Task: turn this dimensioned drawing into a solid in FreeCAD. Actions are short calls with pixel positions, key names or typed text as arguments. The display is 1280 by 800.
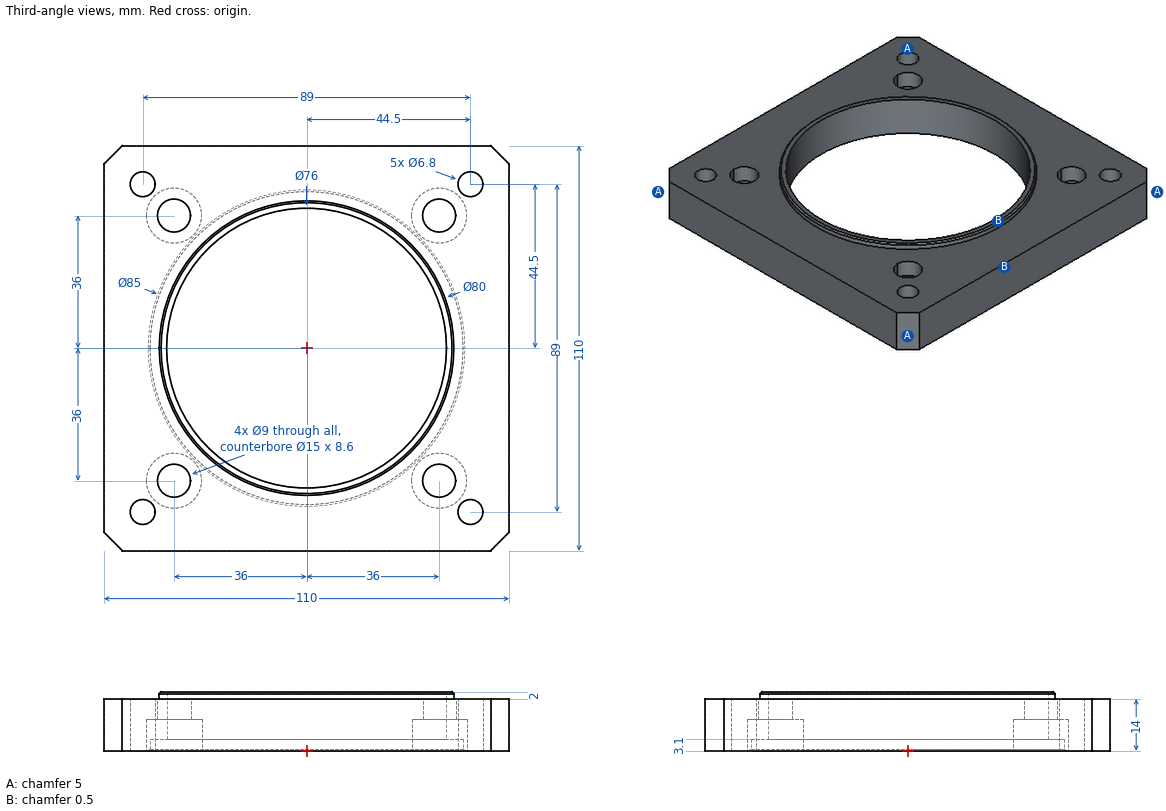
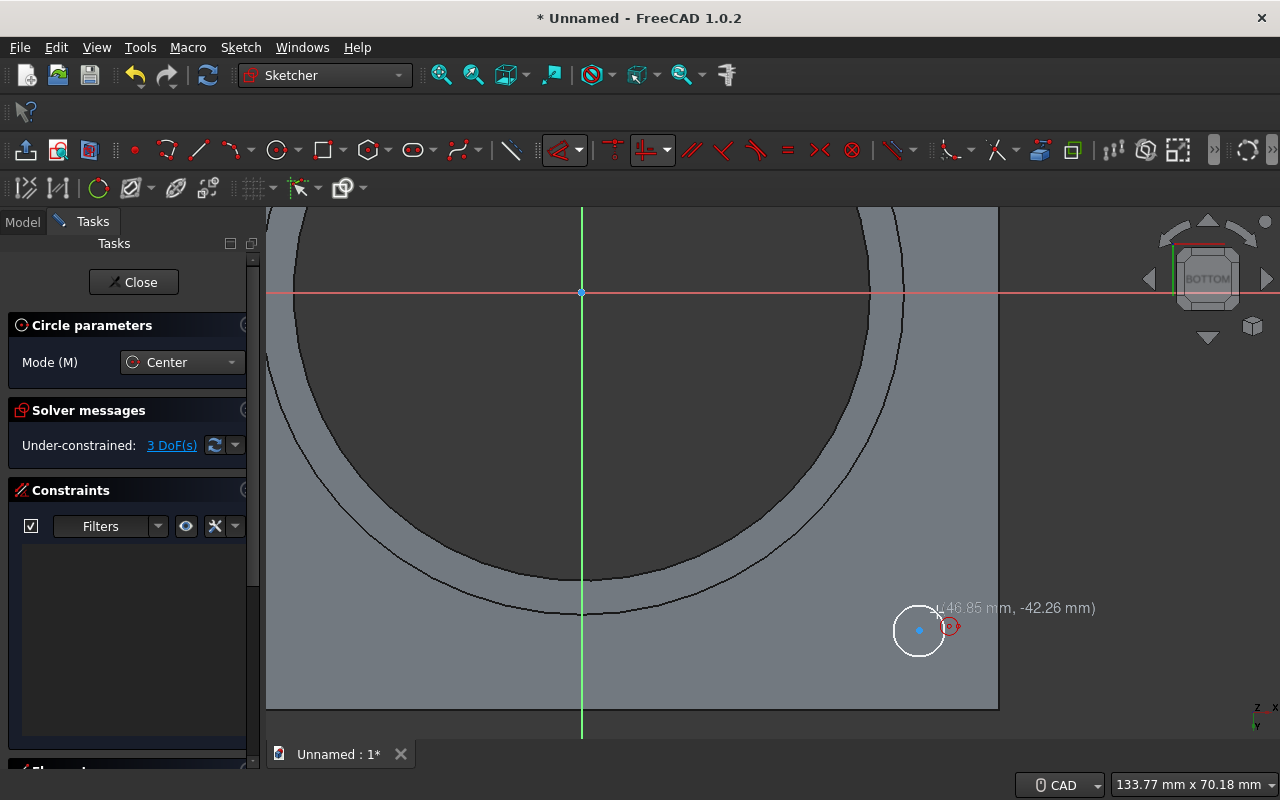
click(582, 293)
click(600, 274)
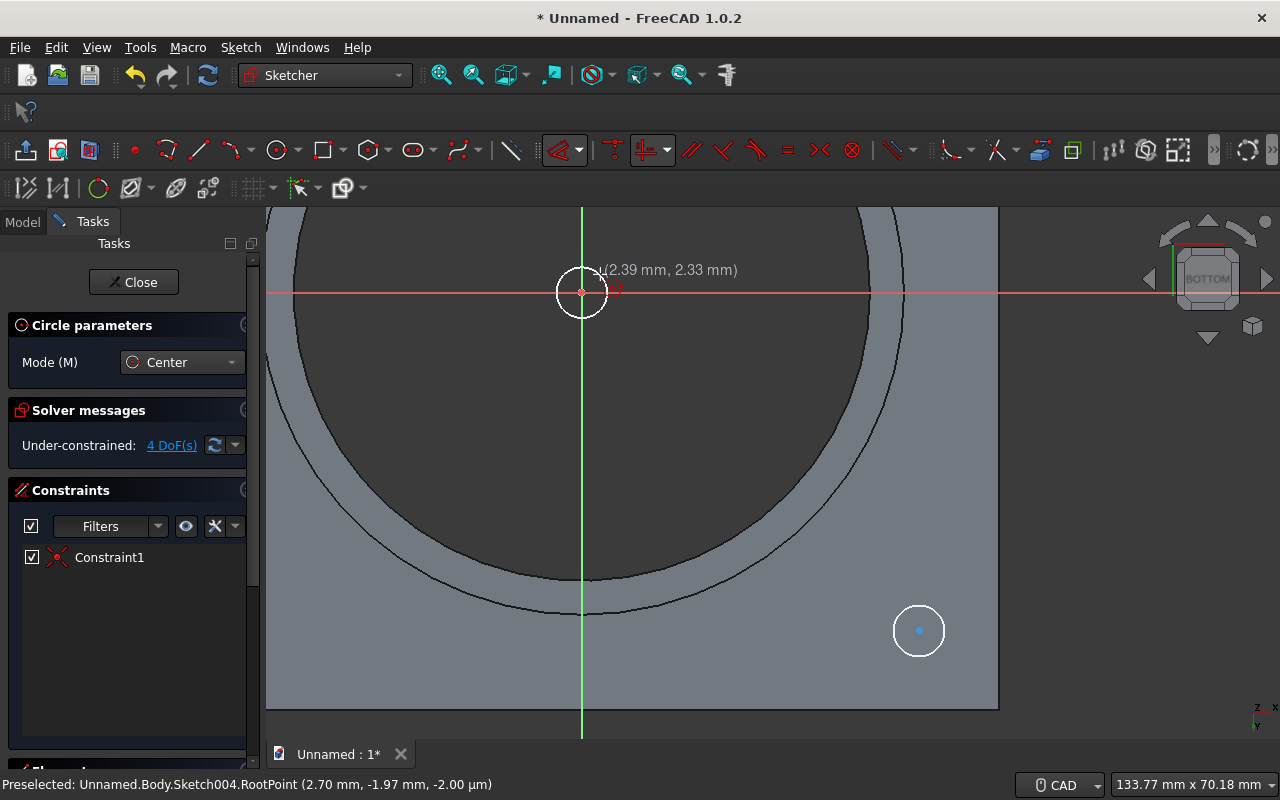
scroll(805, 620, down, 4)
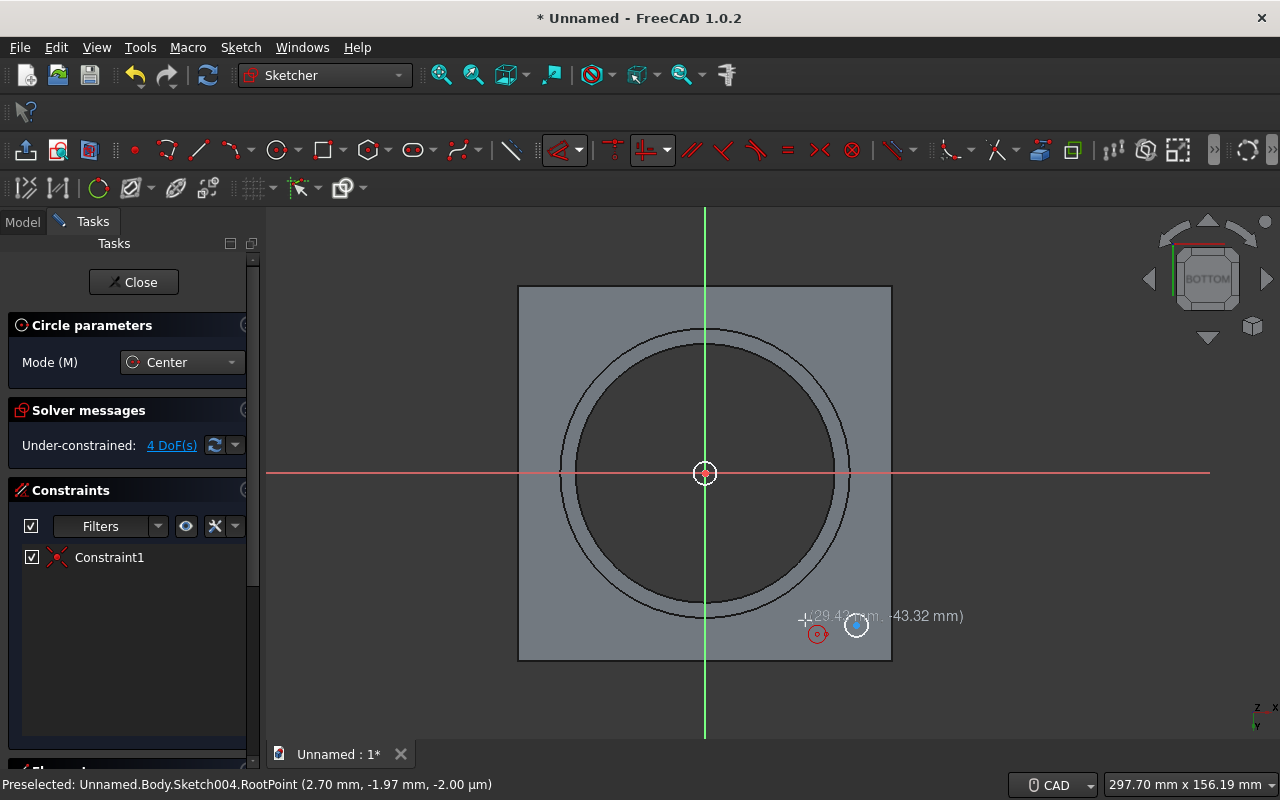
scroll(553, 625, up, 4)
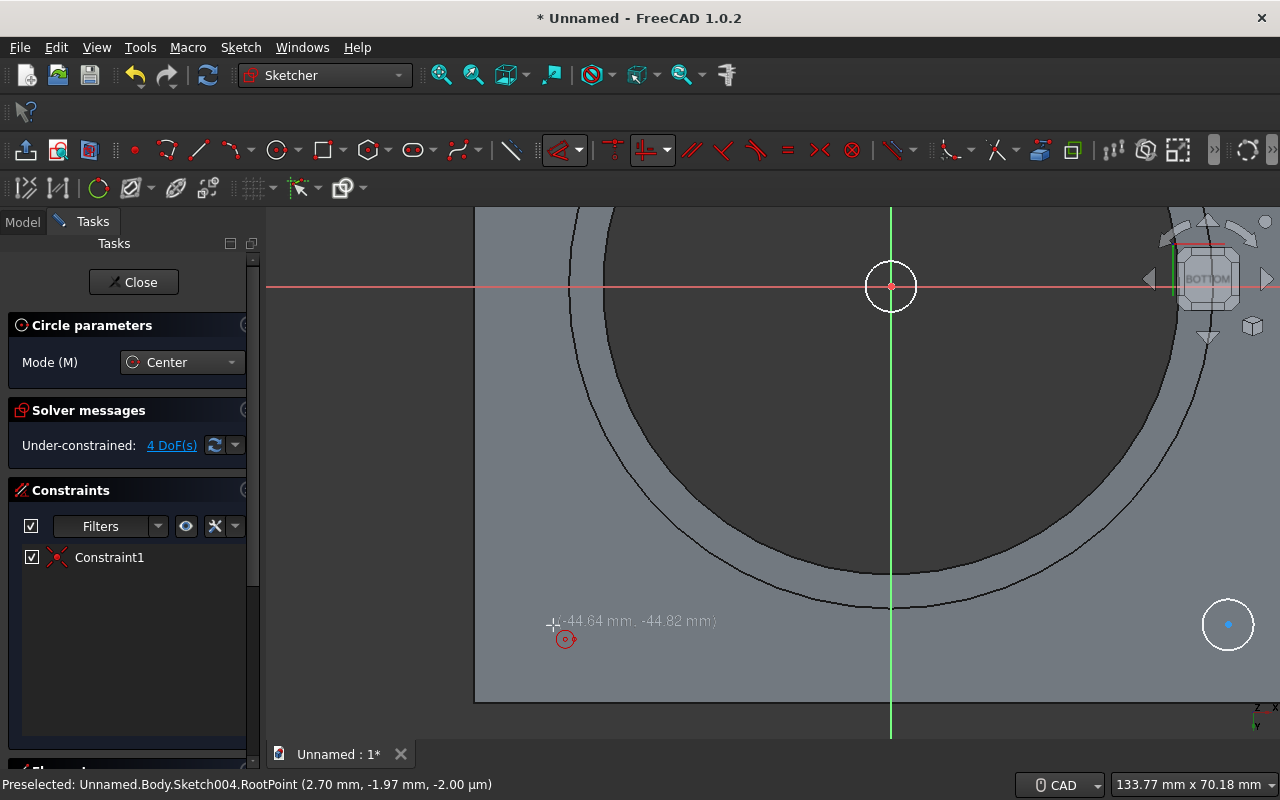
click(554, 624)
click(572, 606)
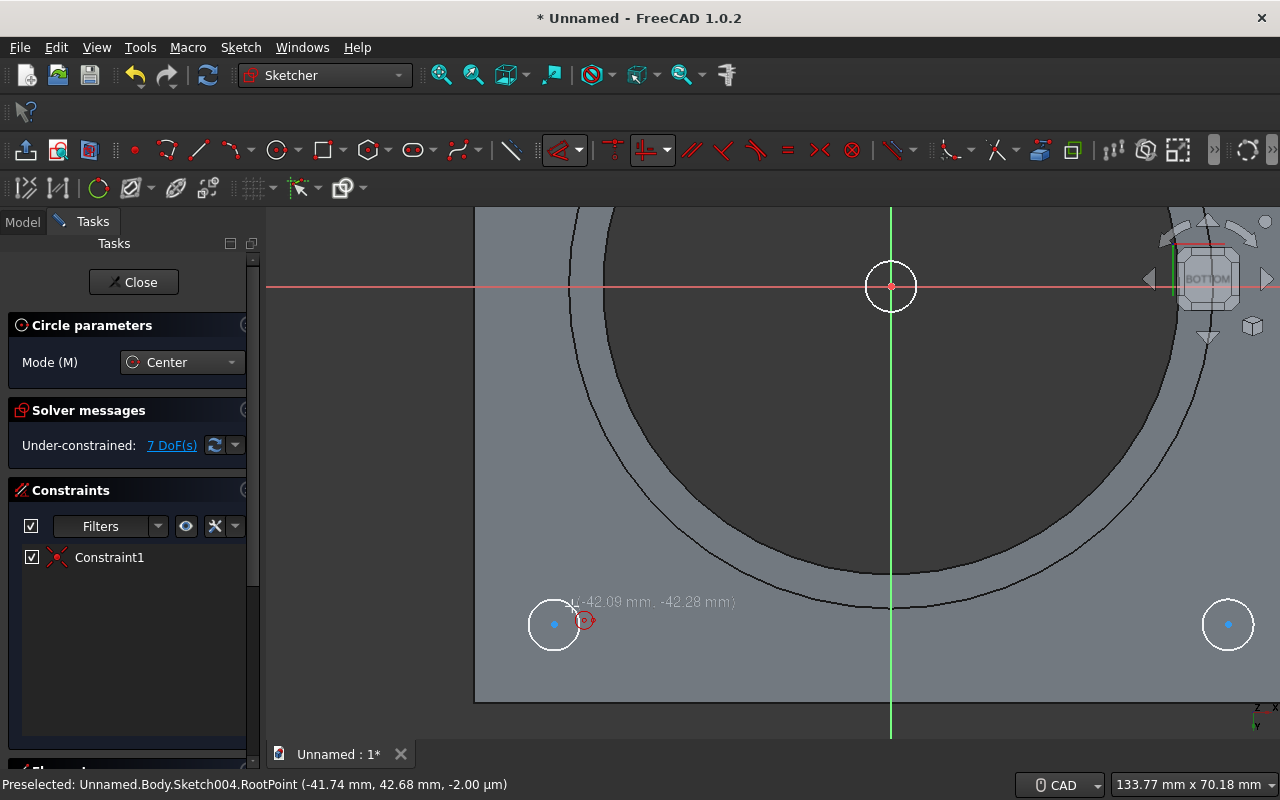
scroll(552, 625, down, 4)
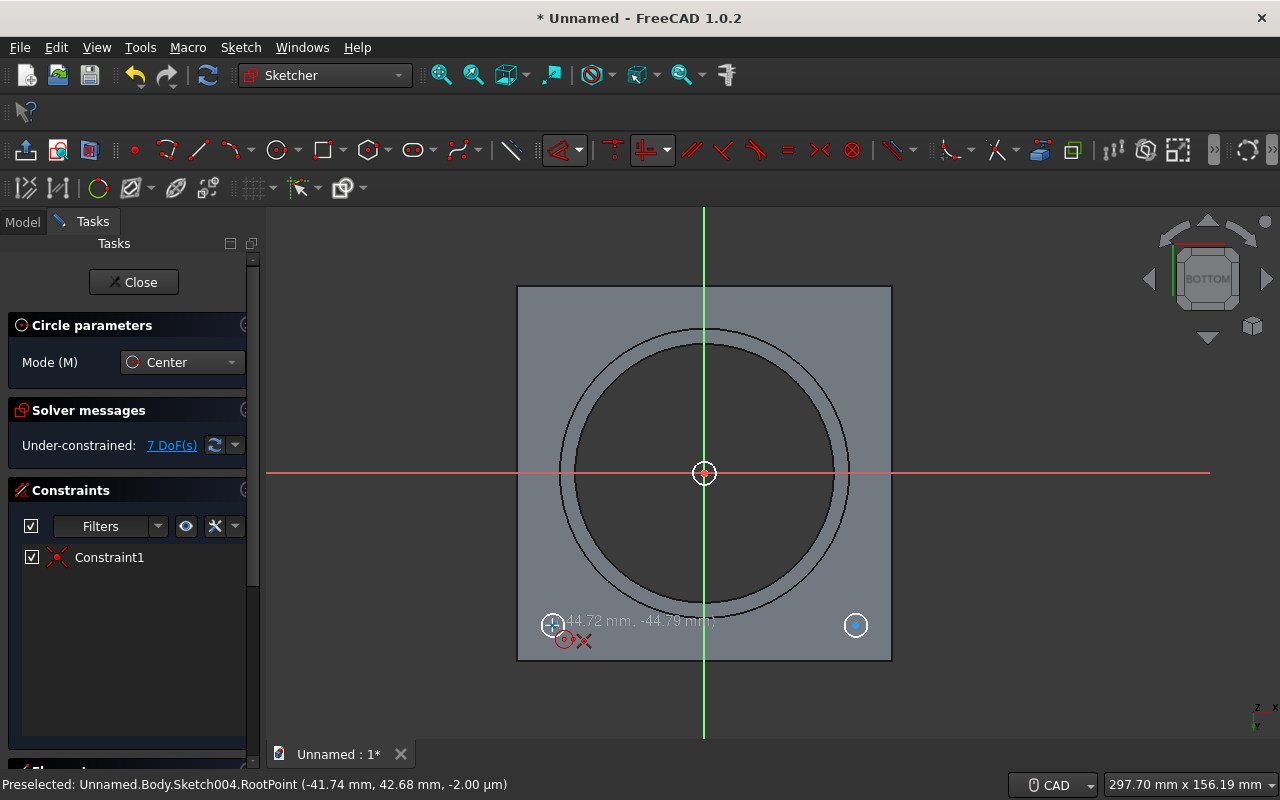
scroll(856, 322, up, 4)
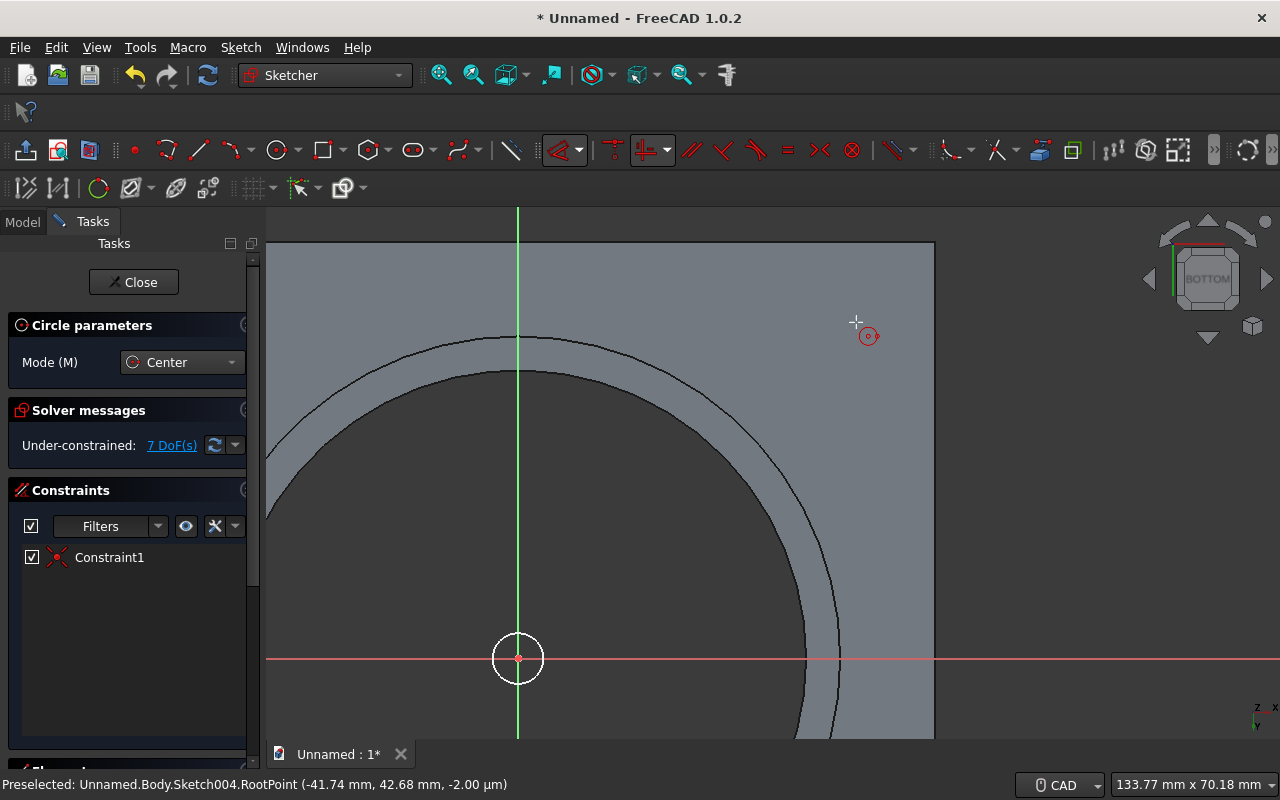
click(855, 321)
click(874, 303)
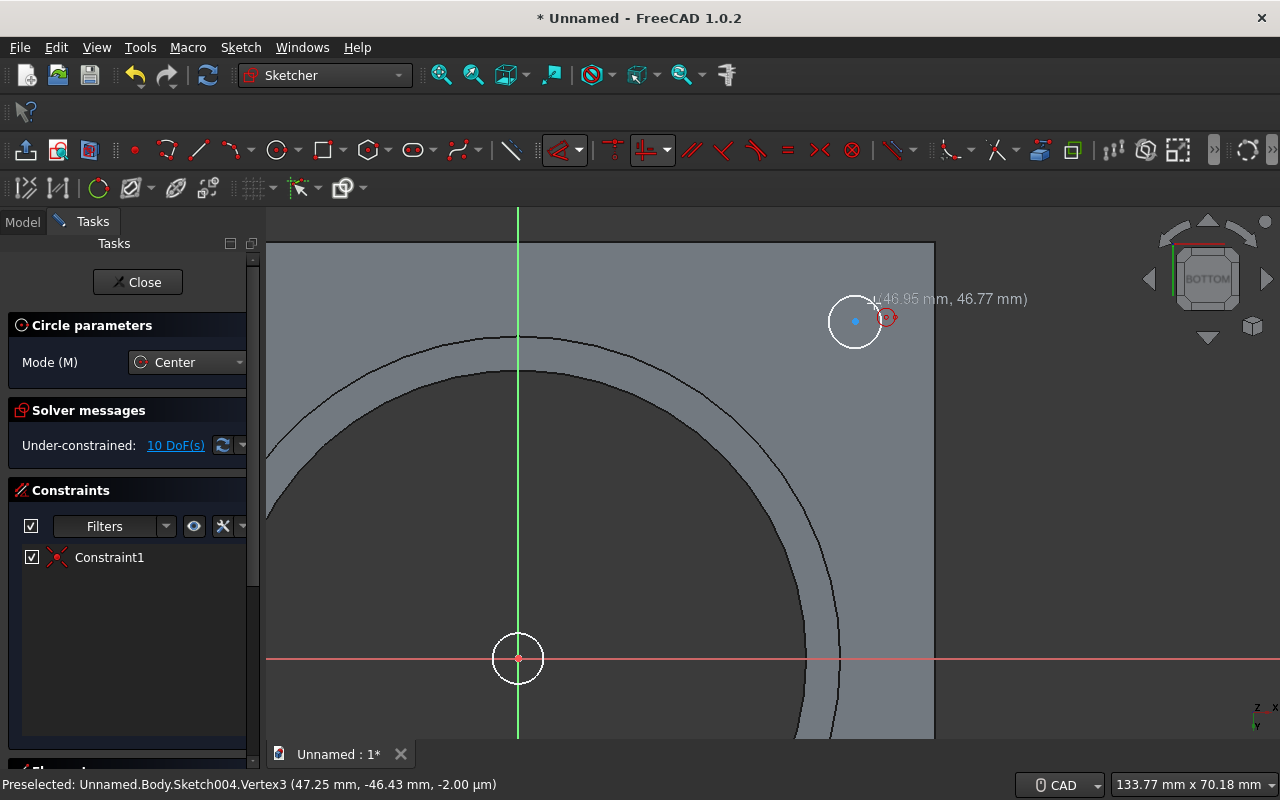
scroll(857, 322, down, 4)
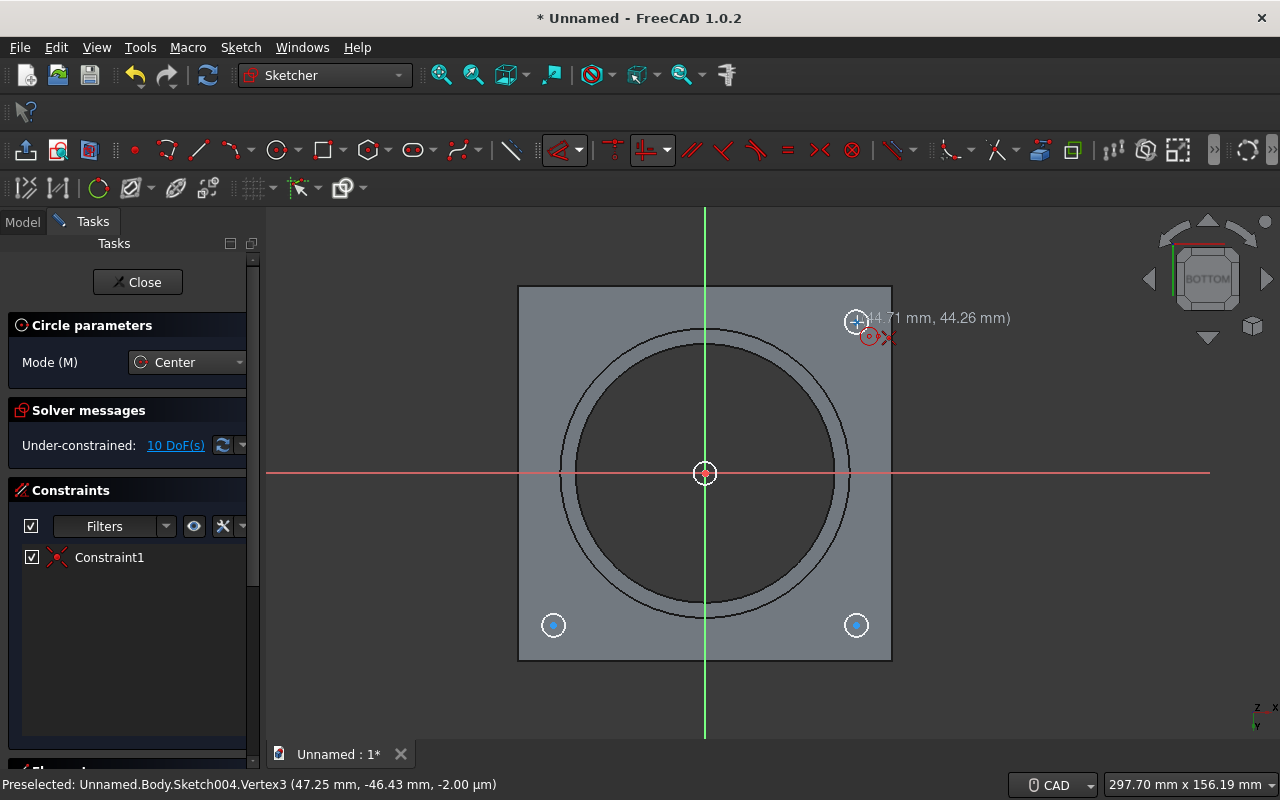
scroll(553, 322, up, 4)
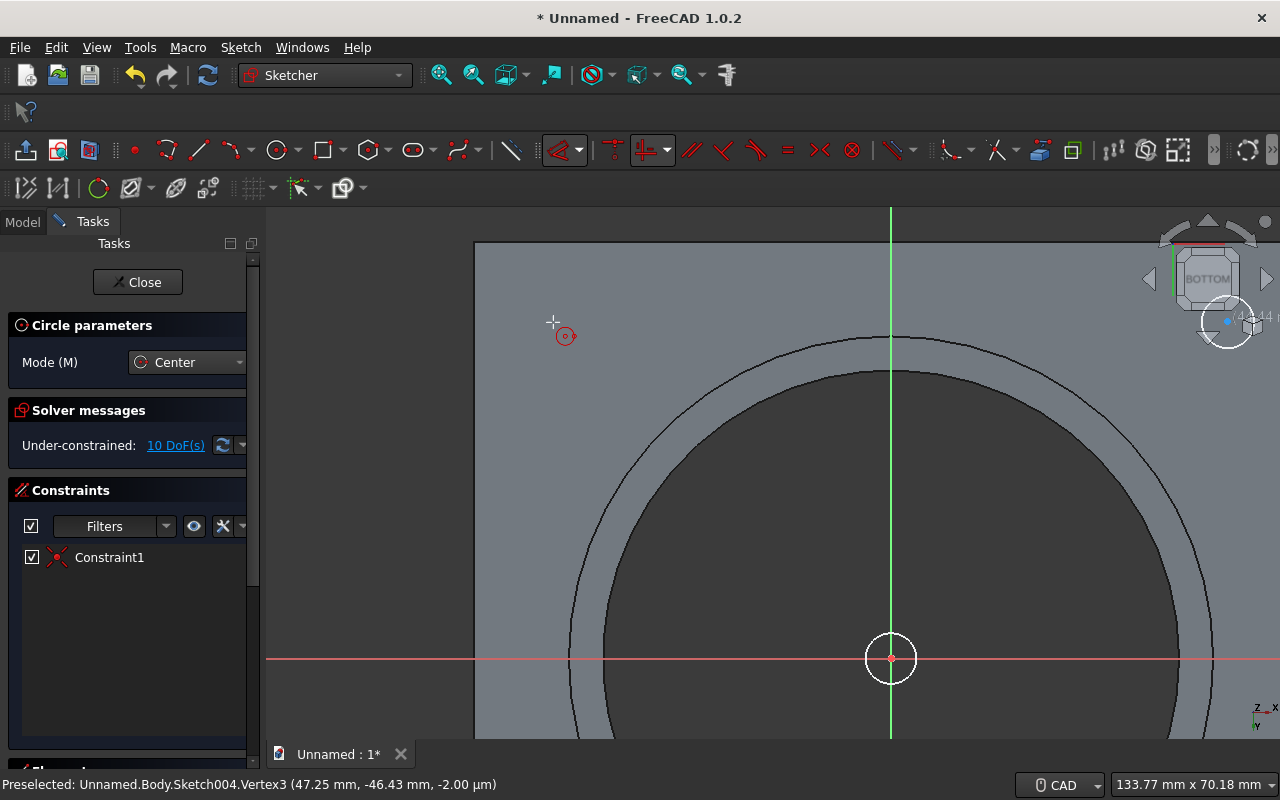
click(554, 321)
click(572, 303)
key(Escape)